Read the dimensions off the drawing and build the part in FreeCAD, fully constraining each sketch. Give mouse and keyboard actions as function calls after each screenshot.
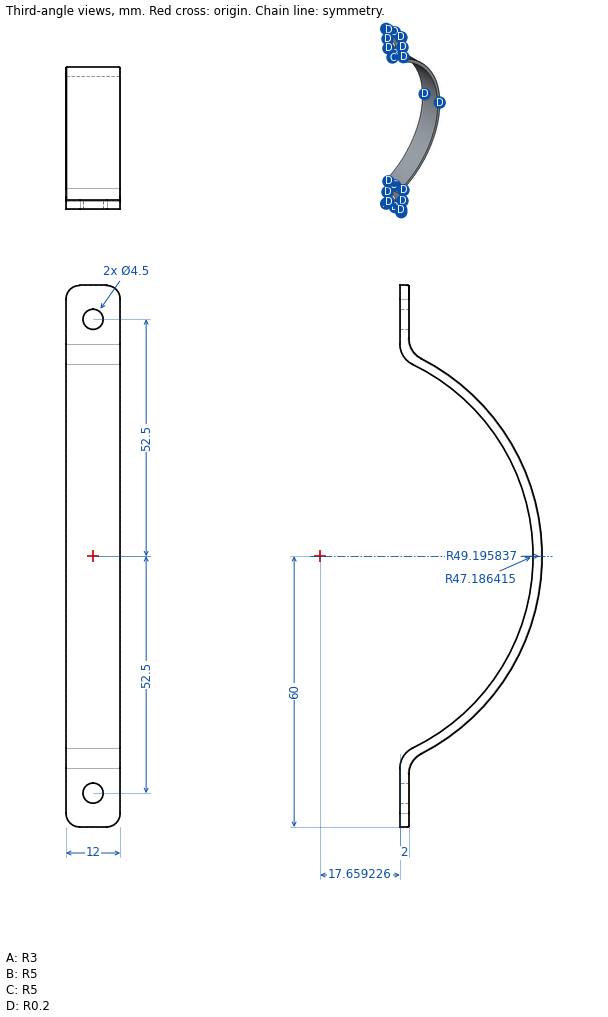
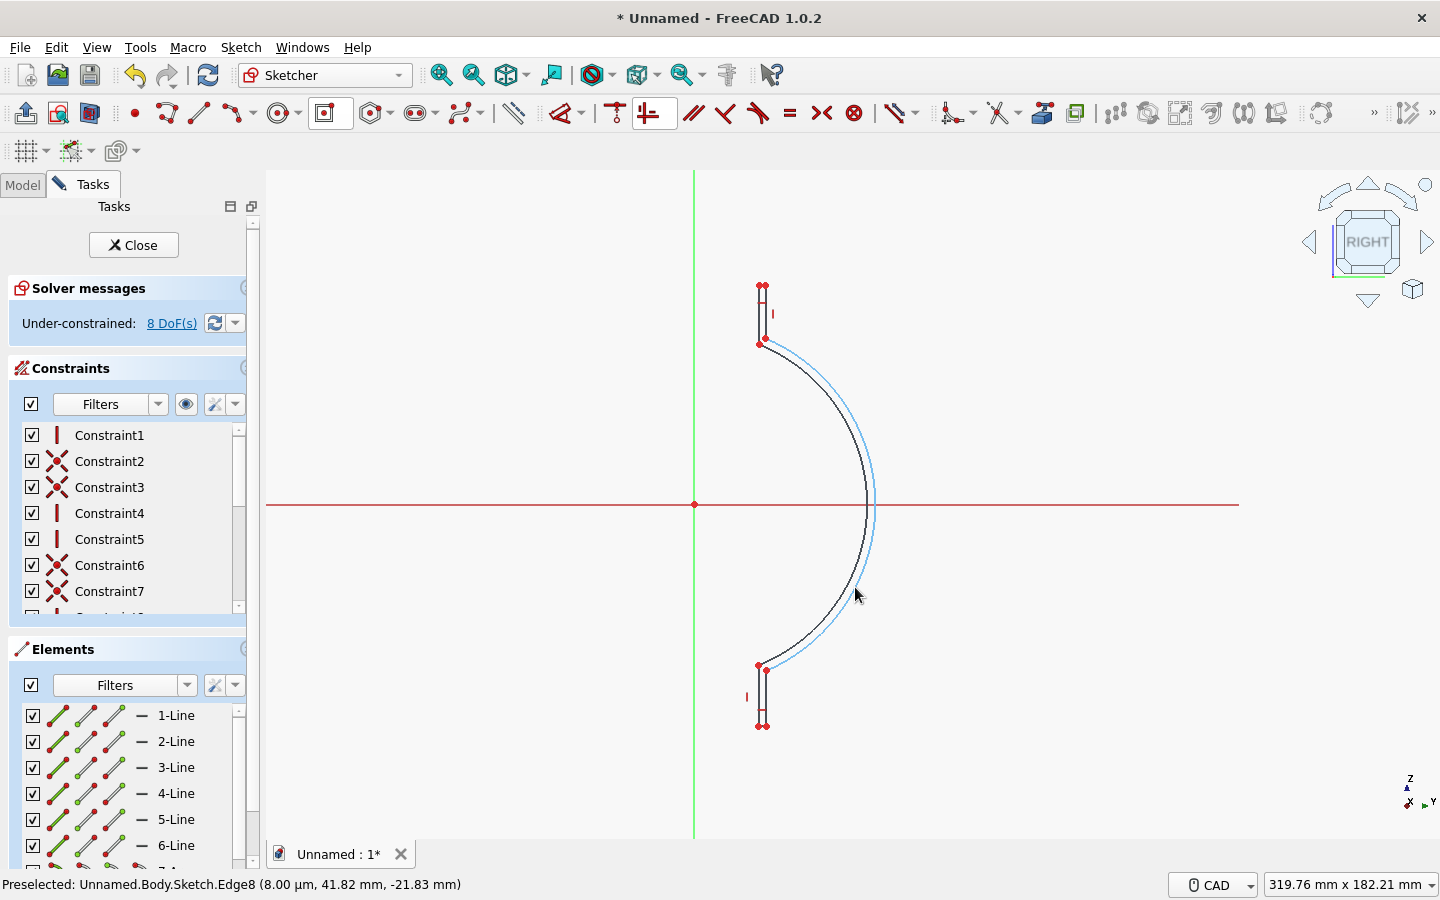
scroll(766, 726, up, 3)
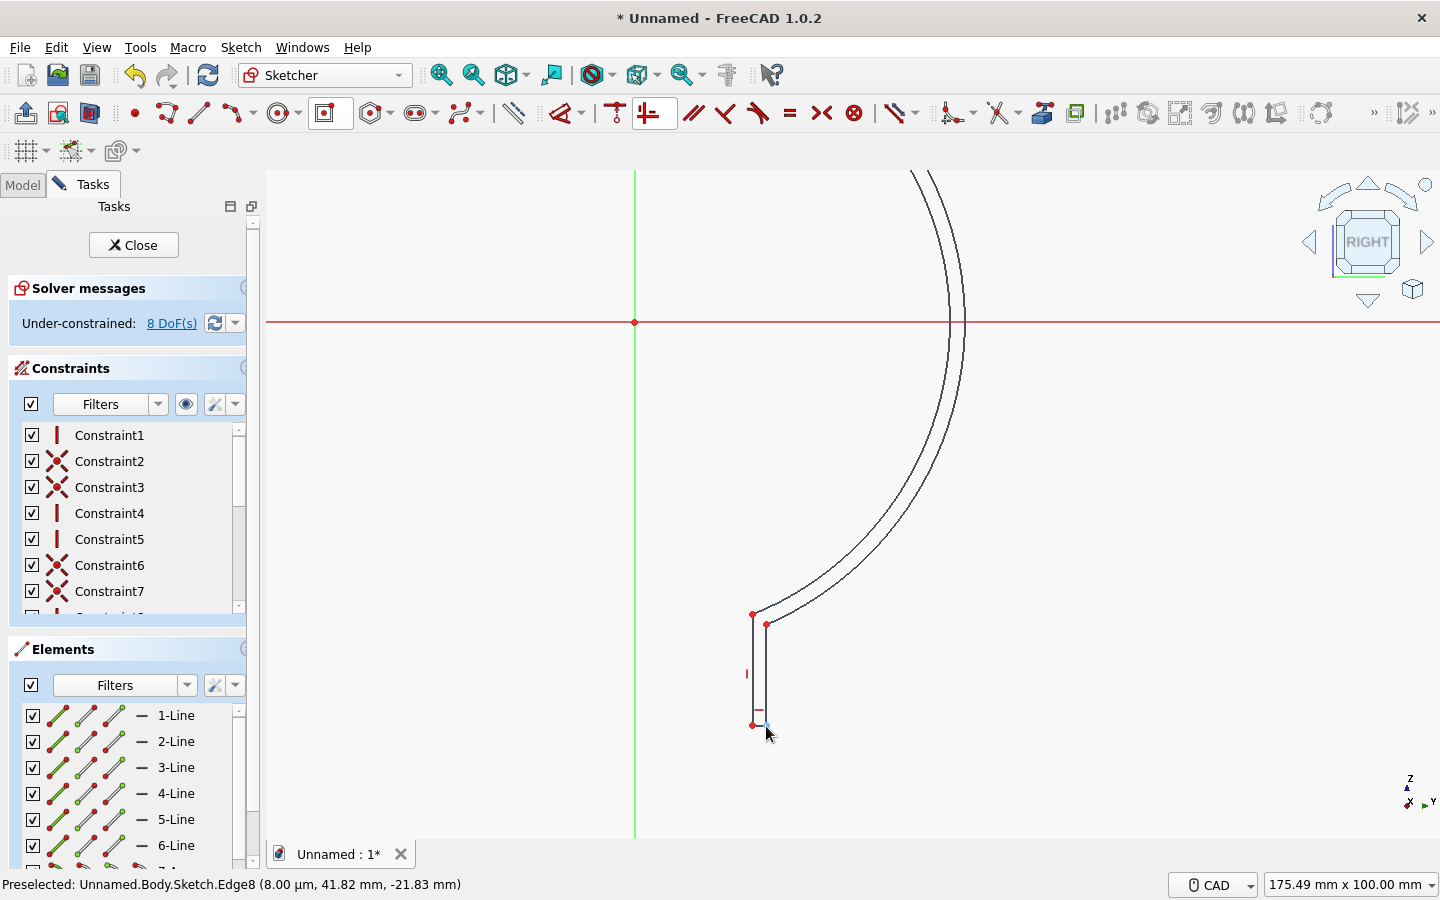
click(766, 726)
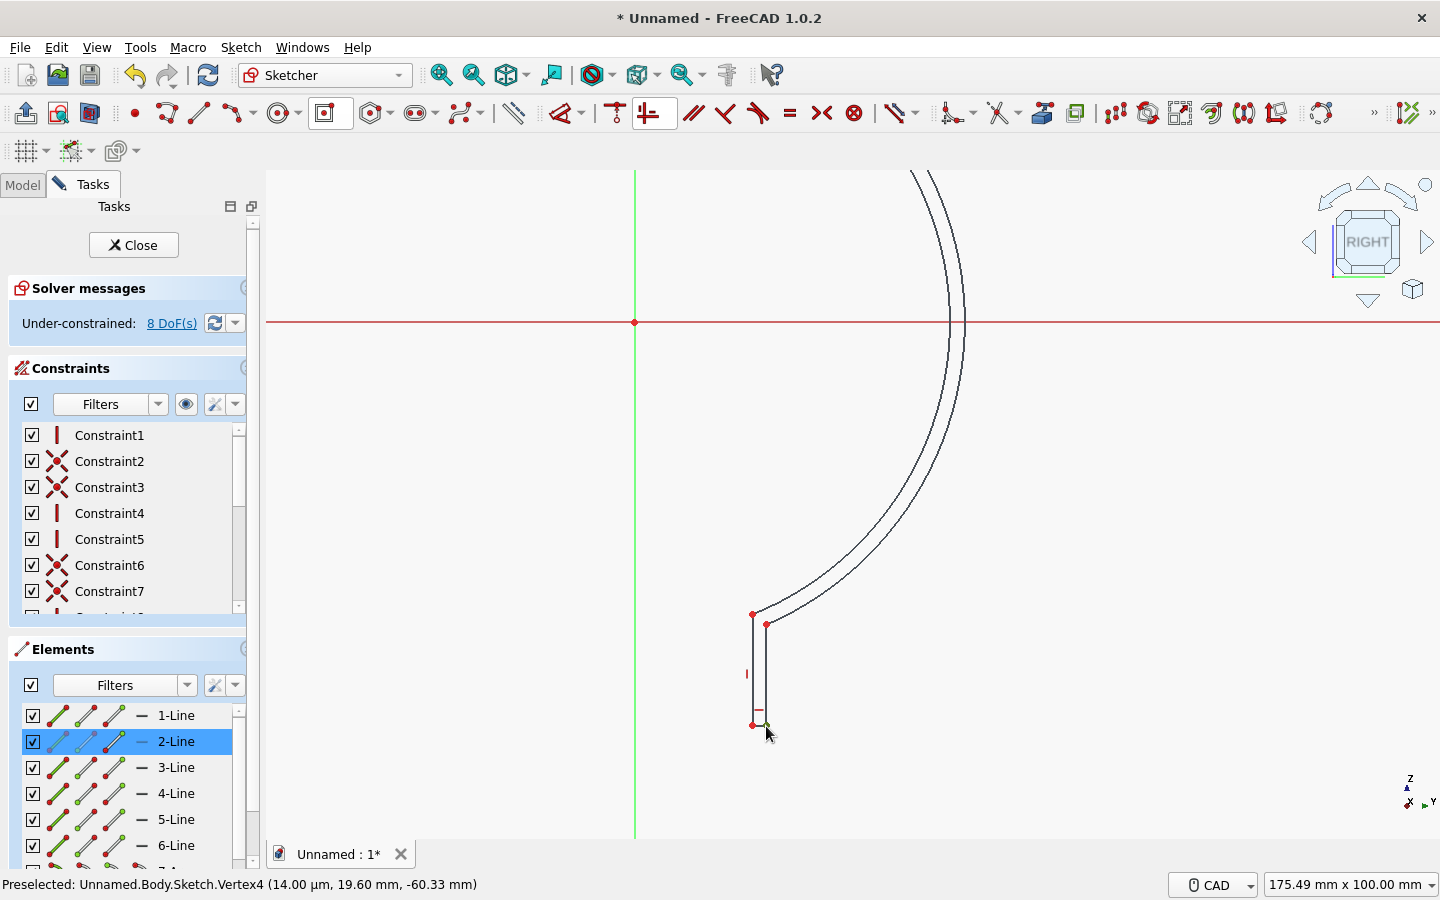
scroll(766, 726, down, 3)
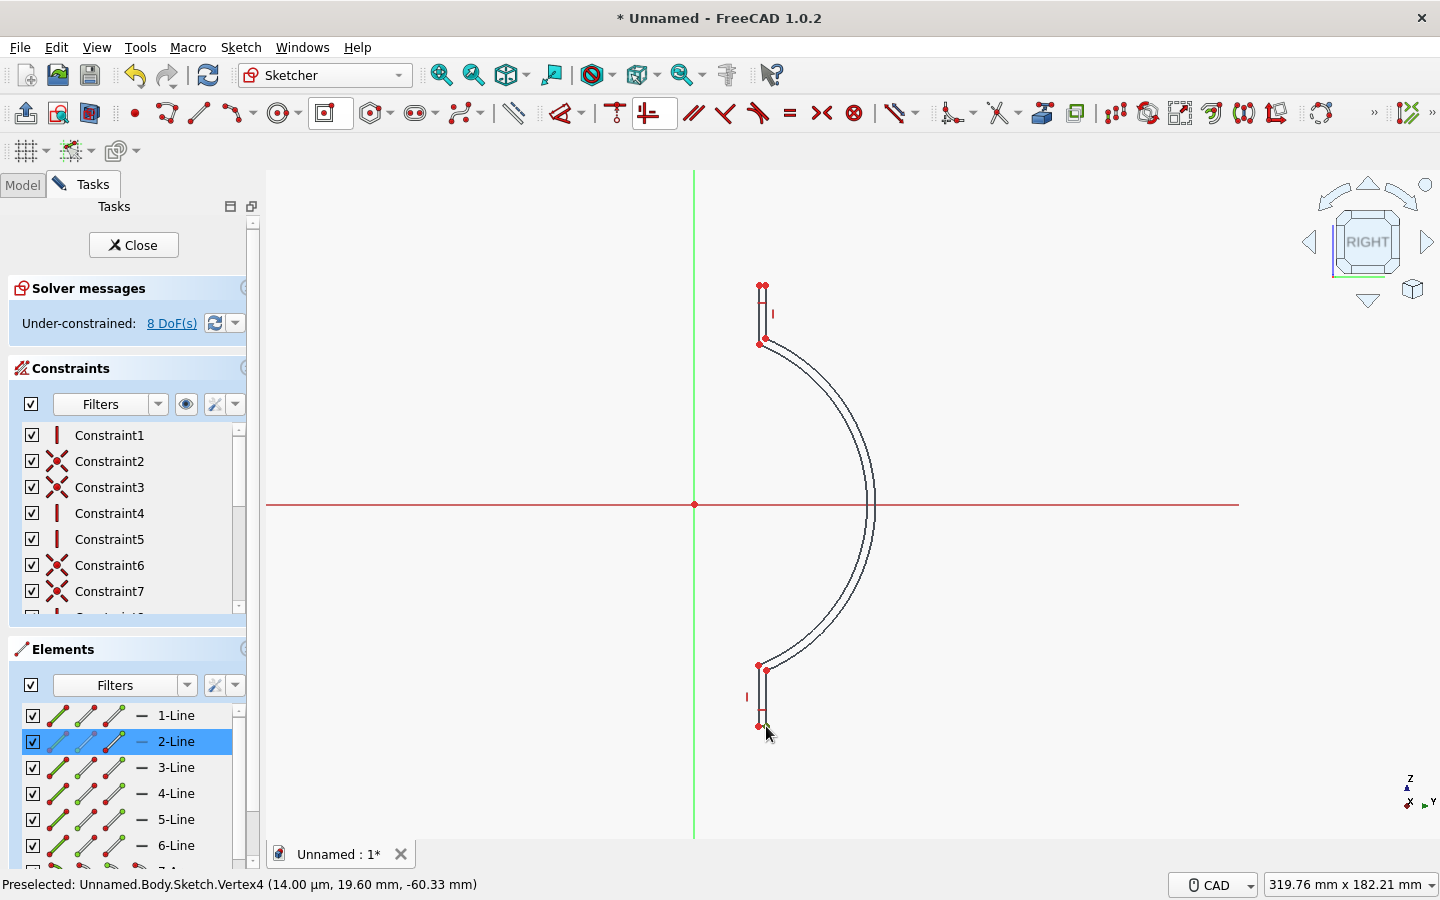
scroll(766, 286, up, 3)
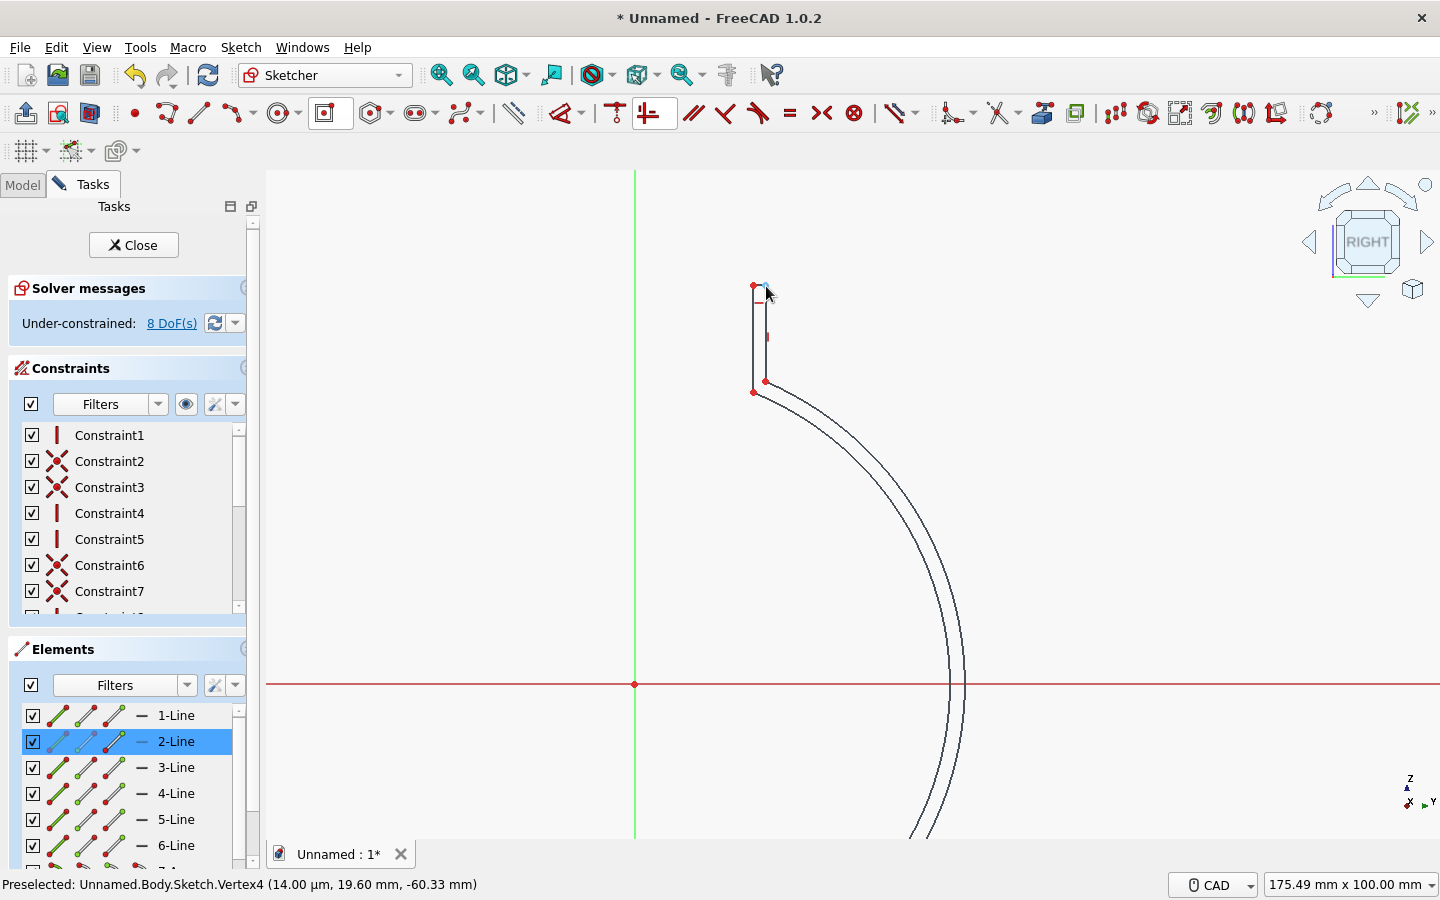
click(766, 285)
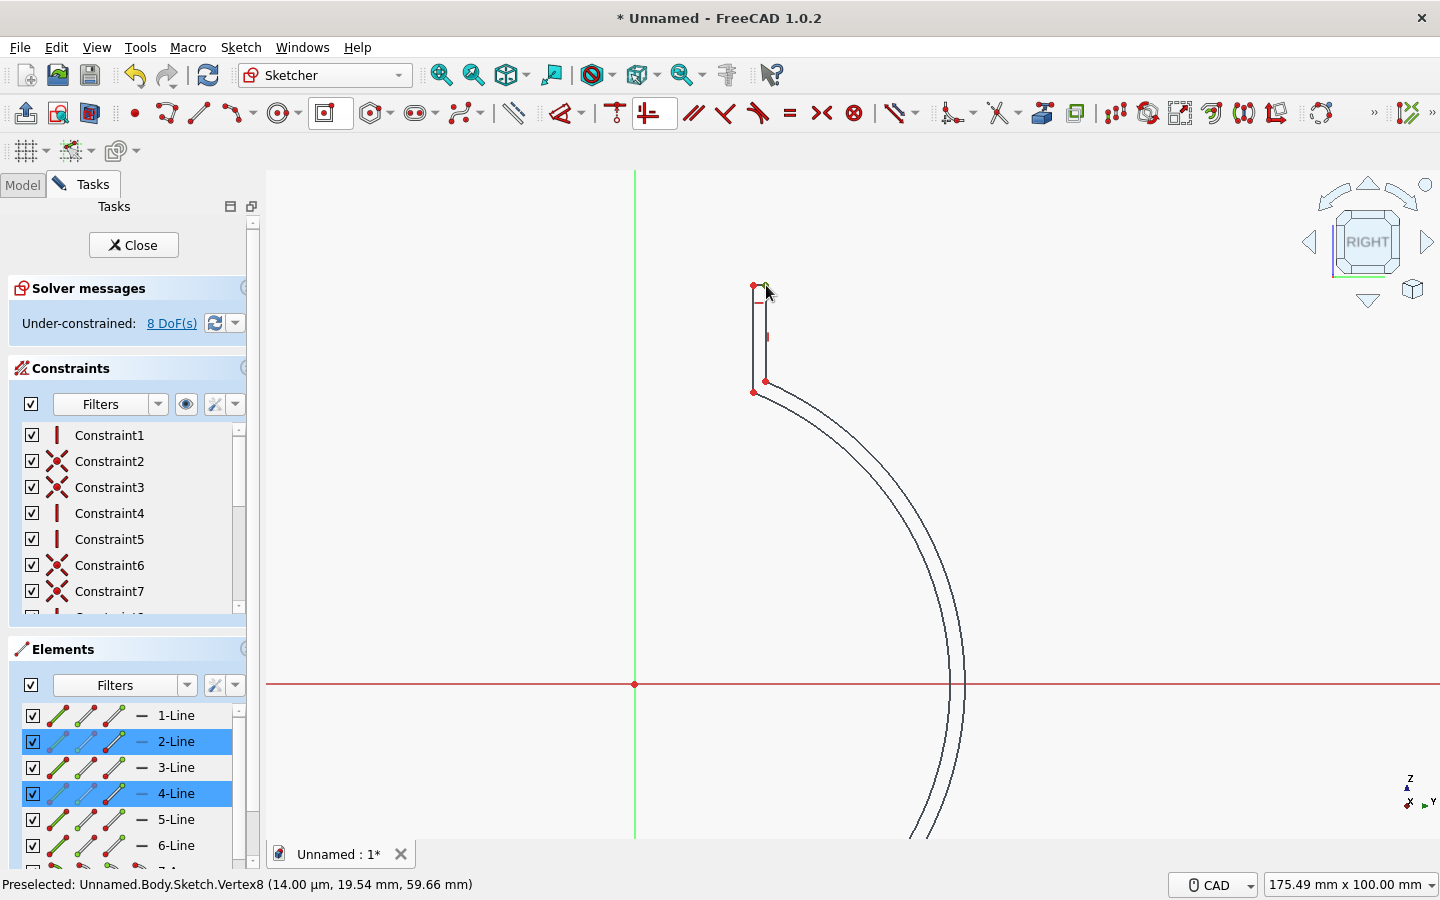
click(364, 684)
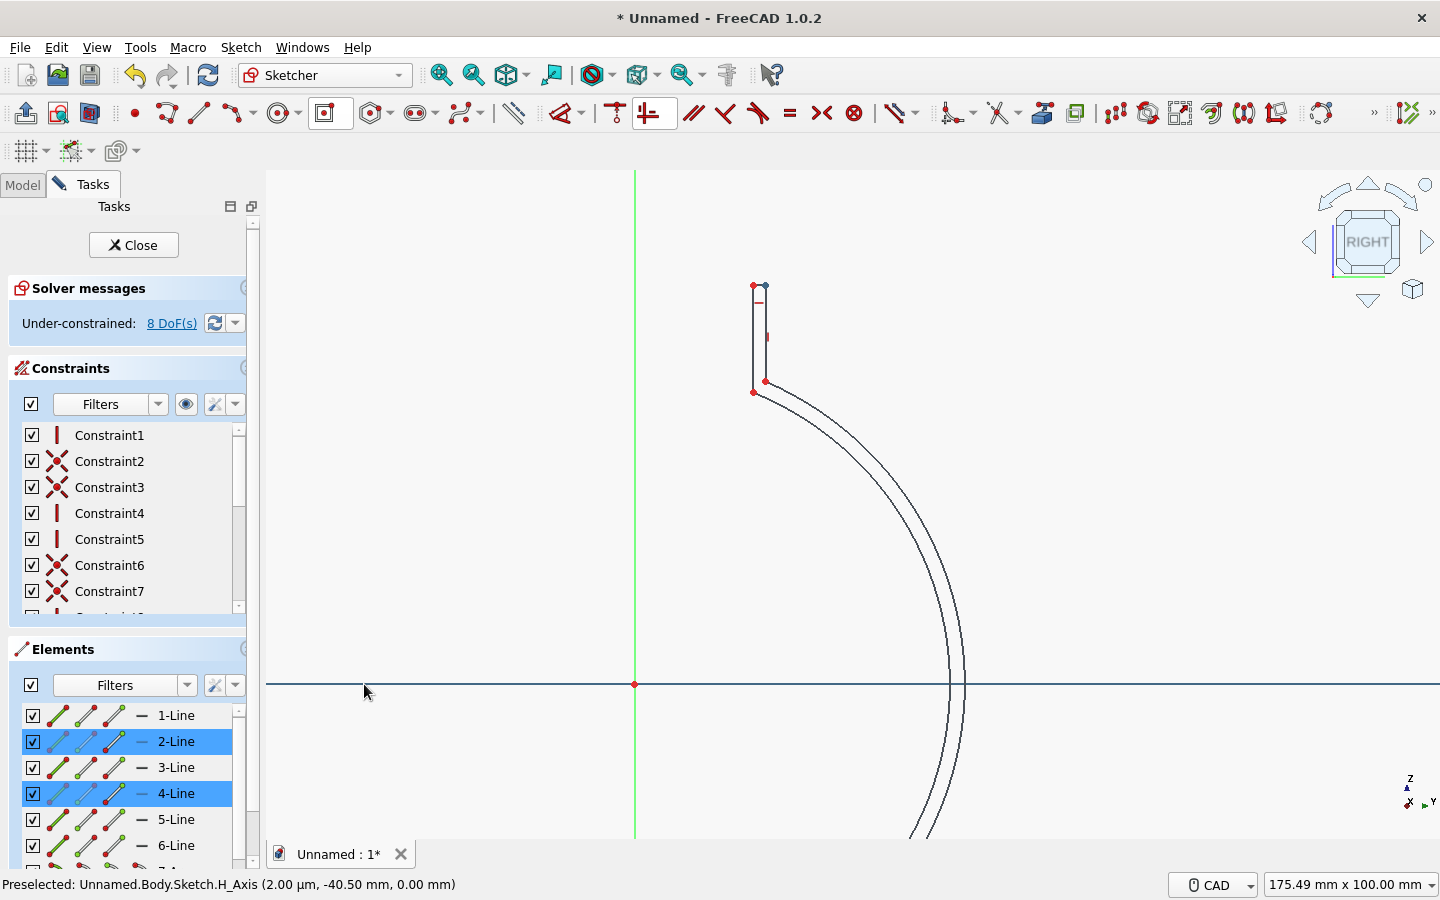
click(822, 114)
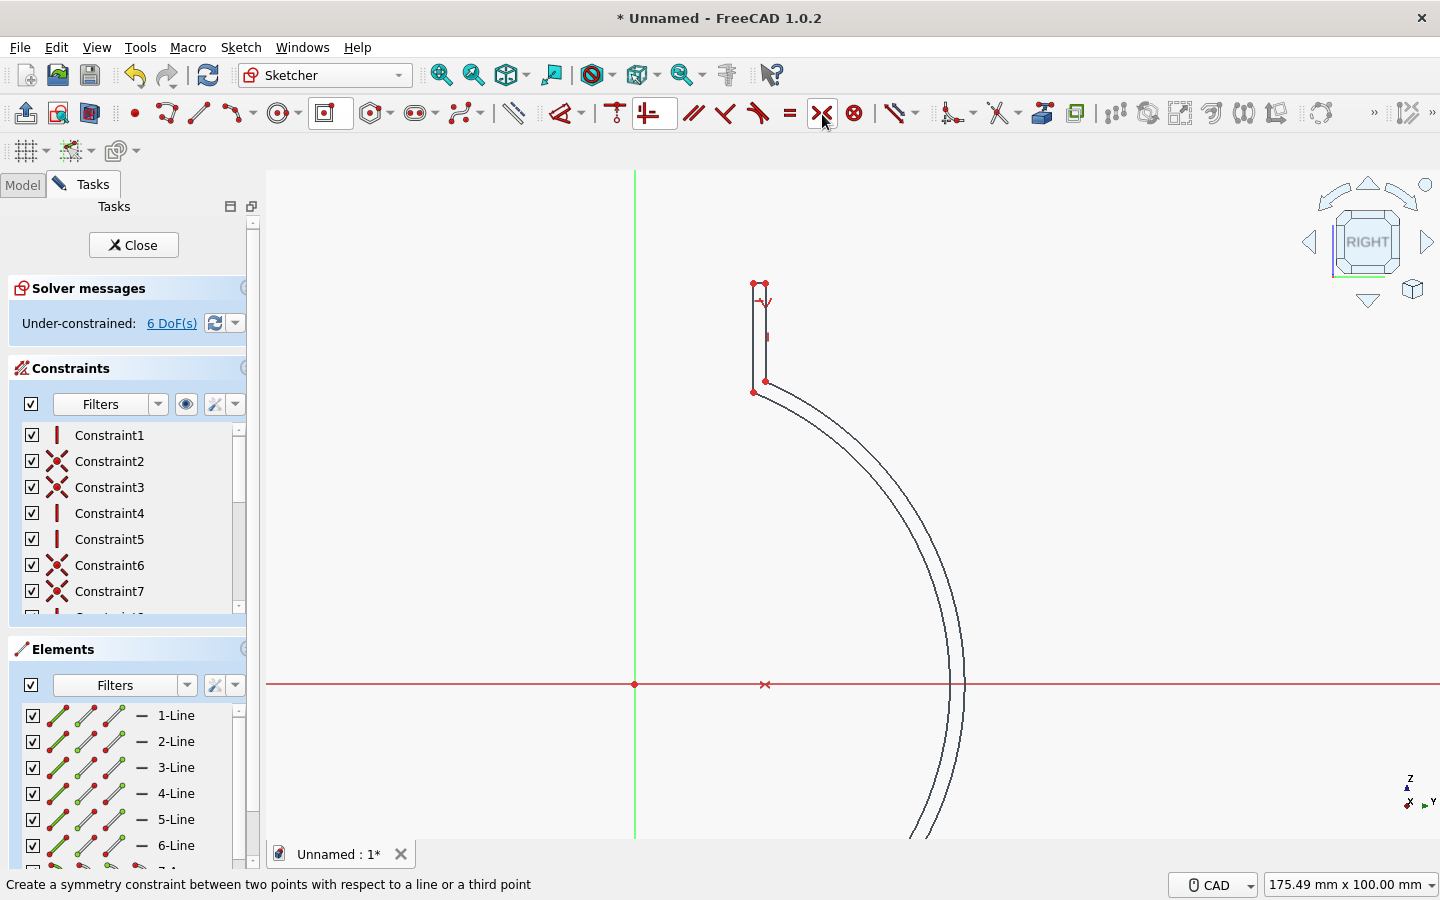
click(560, 114)